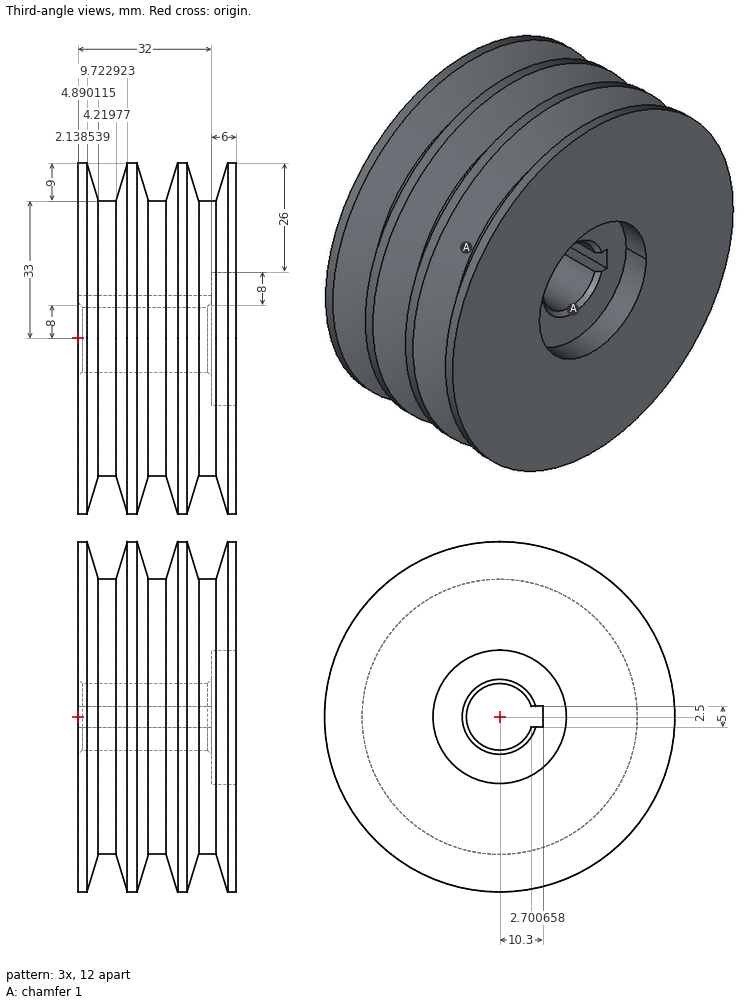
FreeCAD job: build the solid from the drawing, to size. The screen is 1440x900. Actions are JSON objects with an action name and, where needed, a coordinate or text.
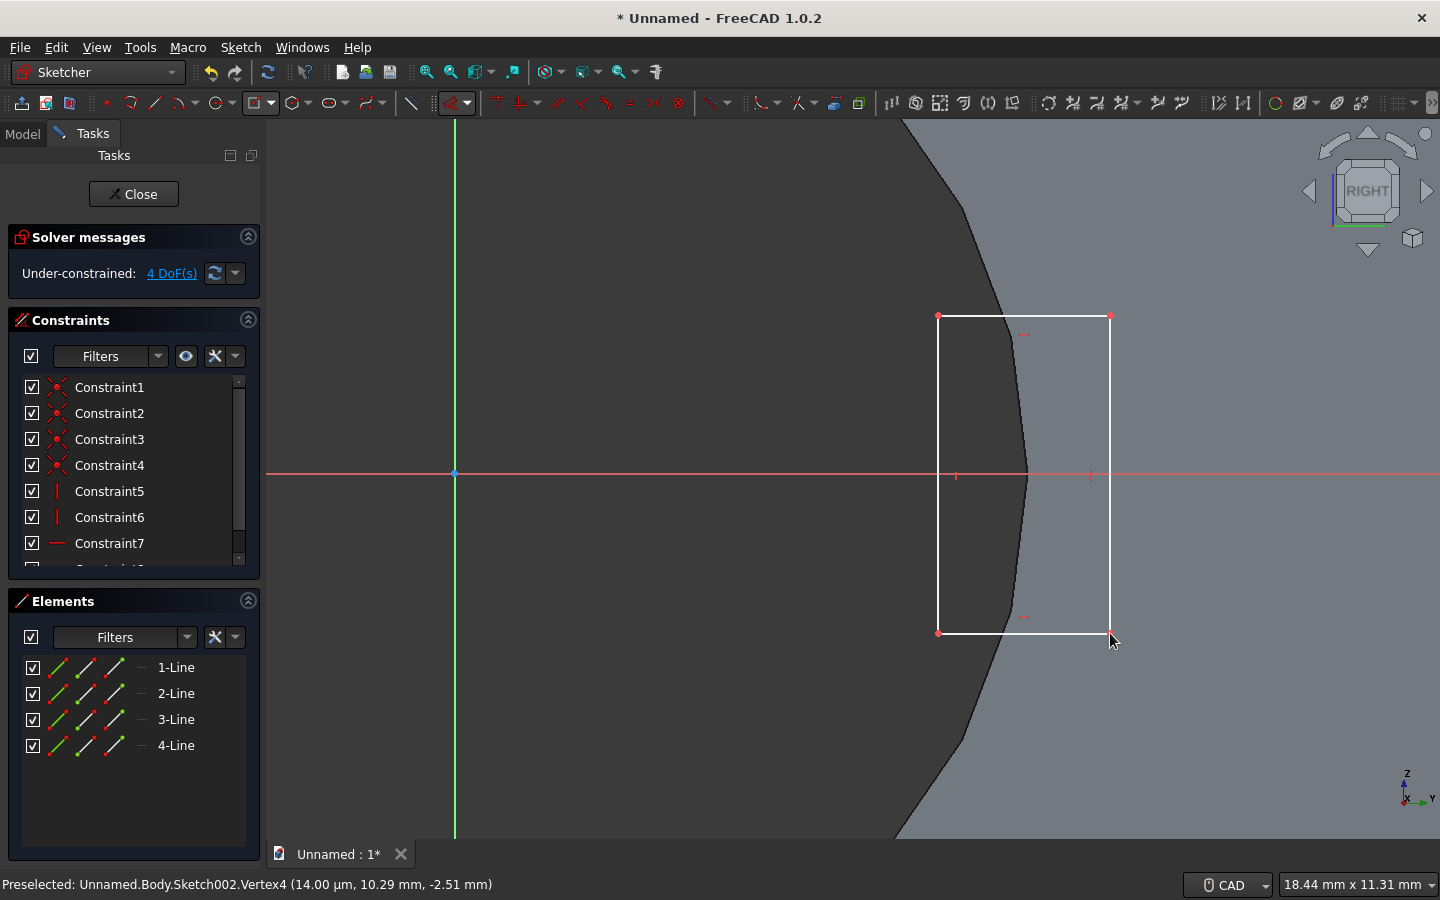
{"action": "key", "text": "d"}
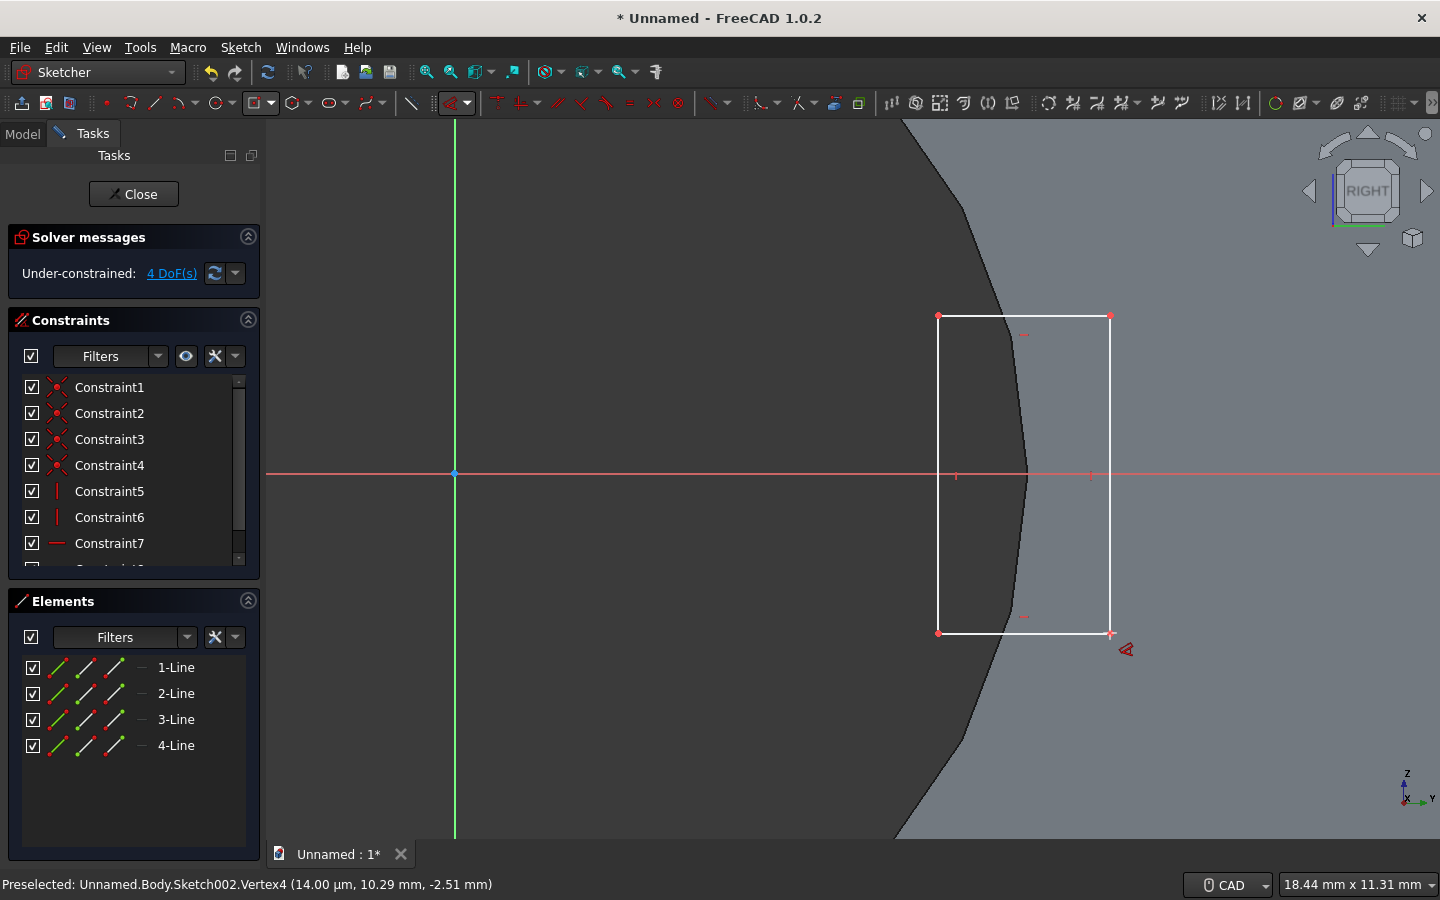
{"action": "left_click", "coordinate": [938, 411]}
{"action": "left_click", "coordinate": [972, 402]}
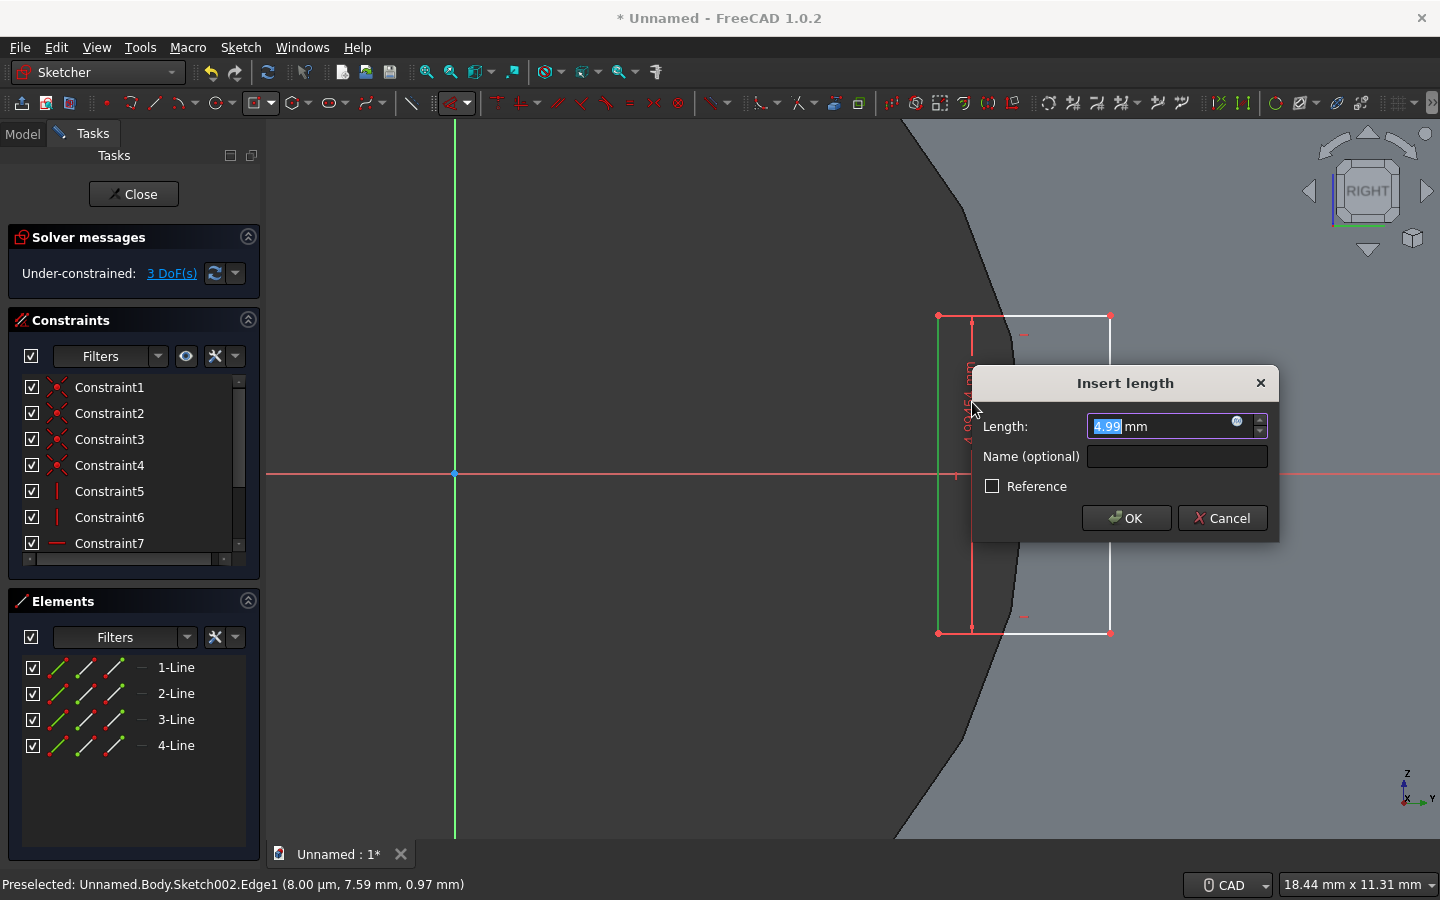
{"action": "type", "text": "5"}
{"action": "key", "text": "Return"}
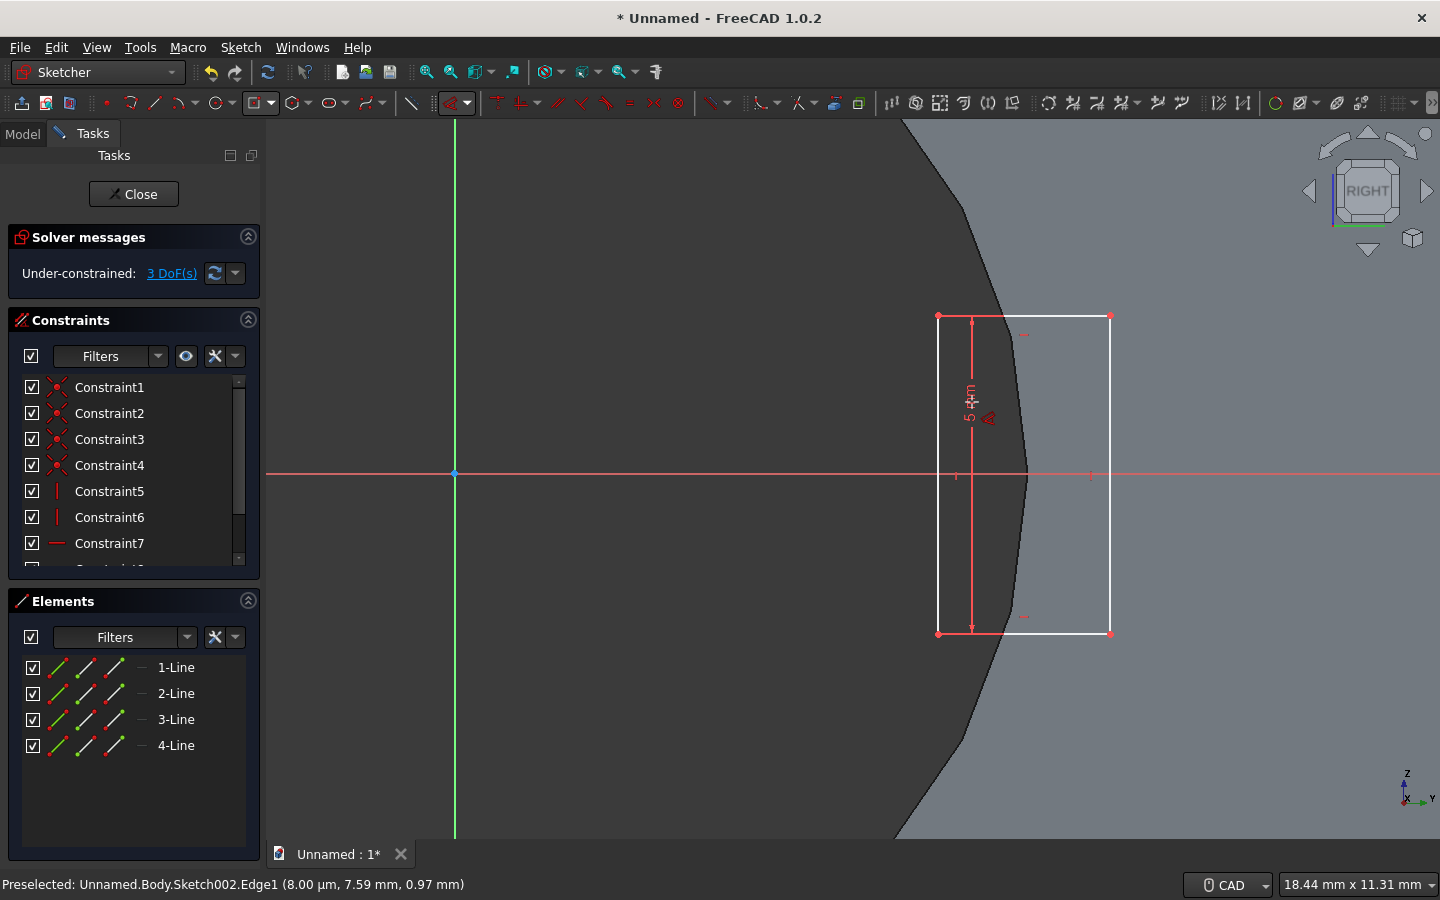
{"action": "left_click", "coordinate": [938, 316]}
{"action": "left_click", "coordinate": [421, 395]}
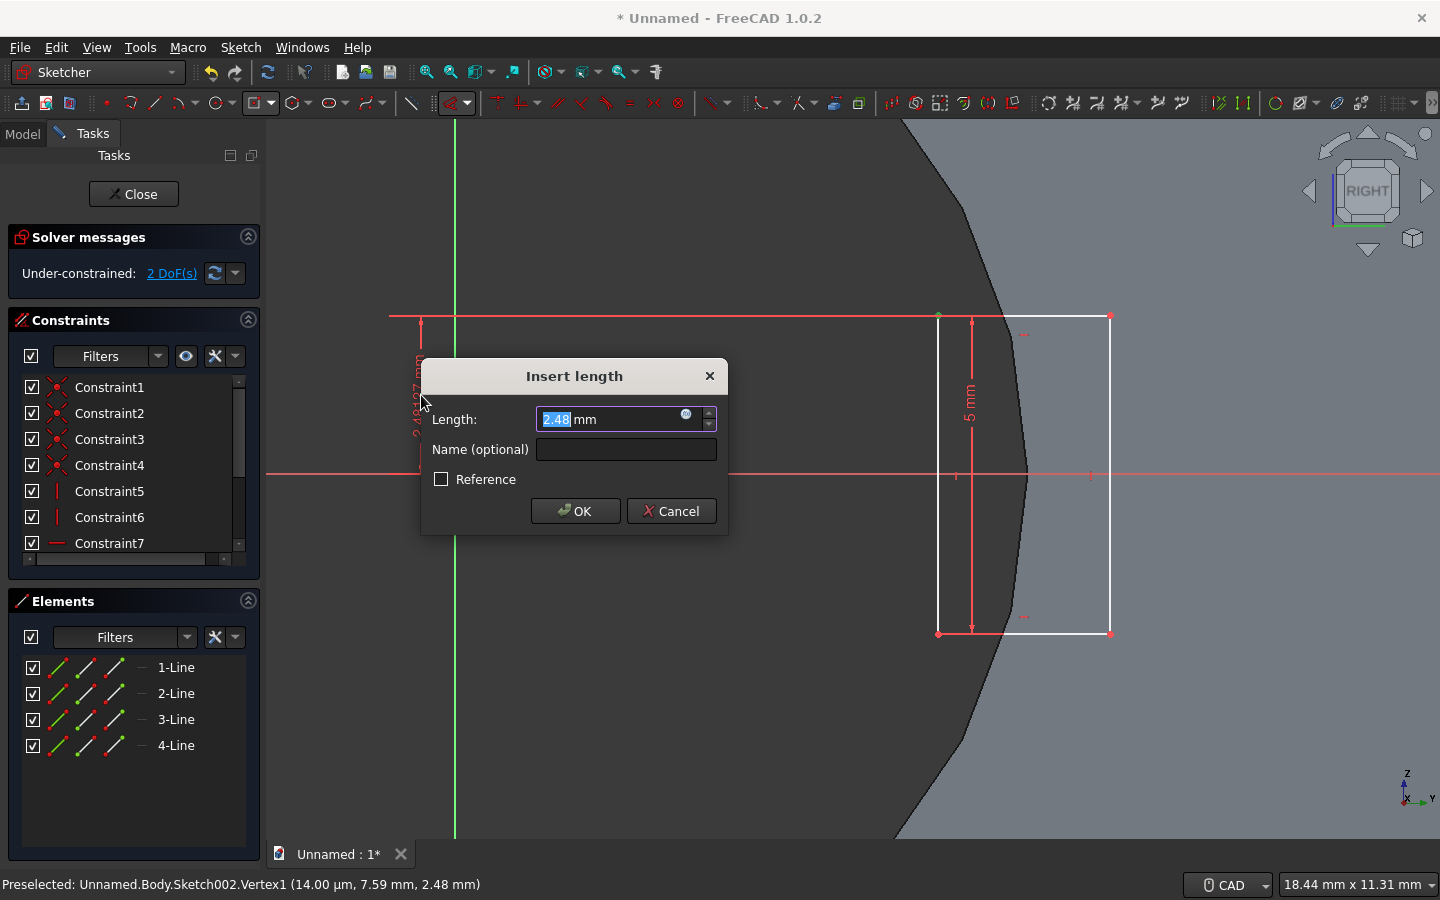
{"action": "type", "text": "2.5"}
{"action": "key", "text": "Return"}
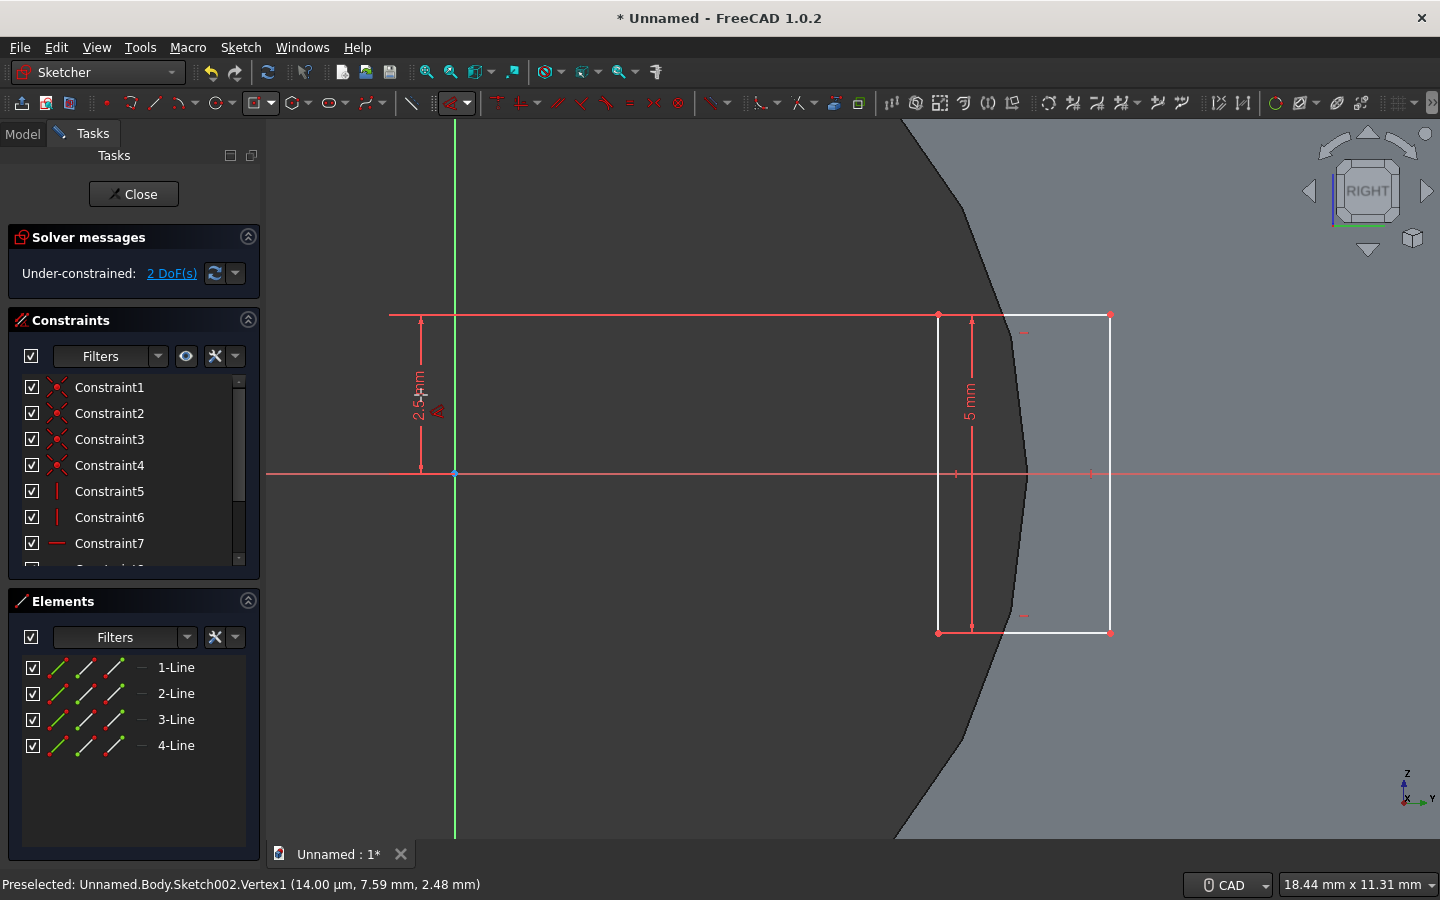
{"action": "left_click", "coordinate": [1110, 633]}
{"action": "left_click", "coordinate": [782, 667]}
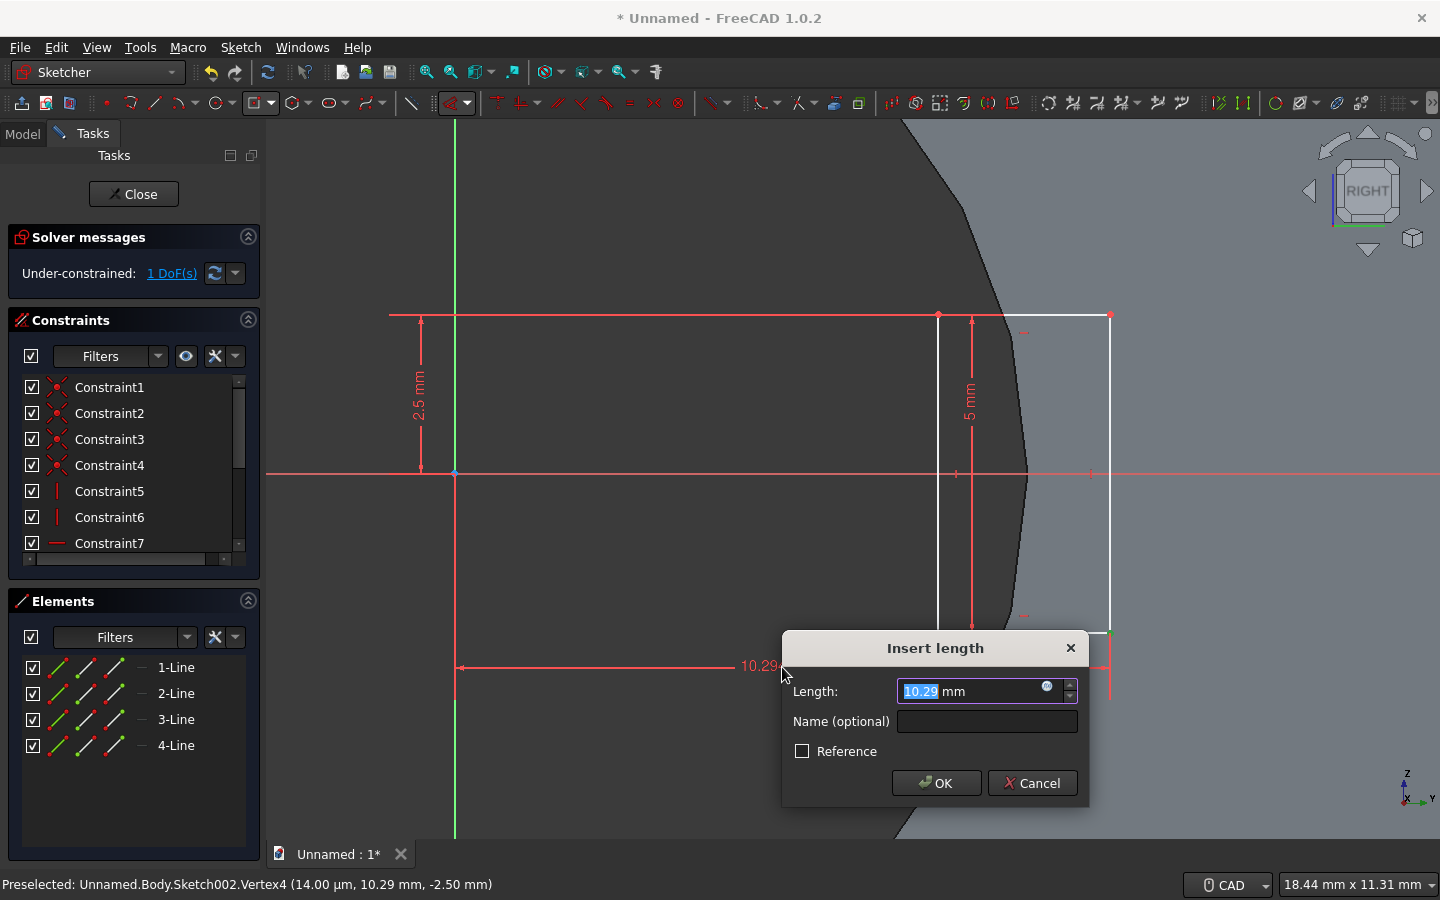
{"action": "type", "text": "10.3"}
{"action": "key", "text": "Return"}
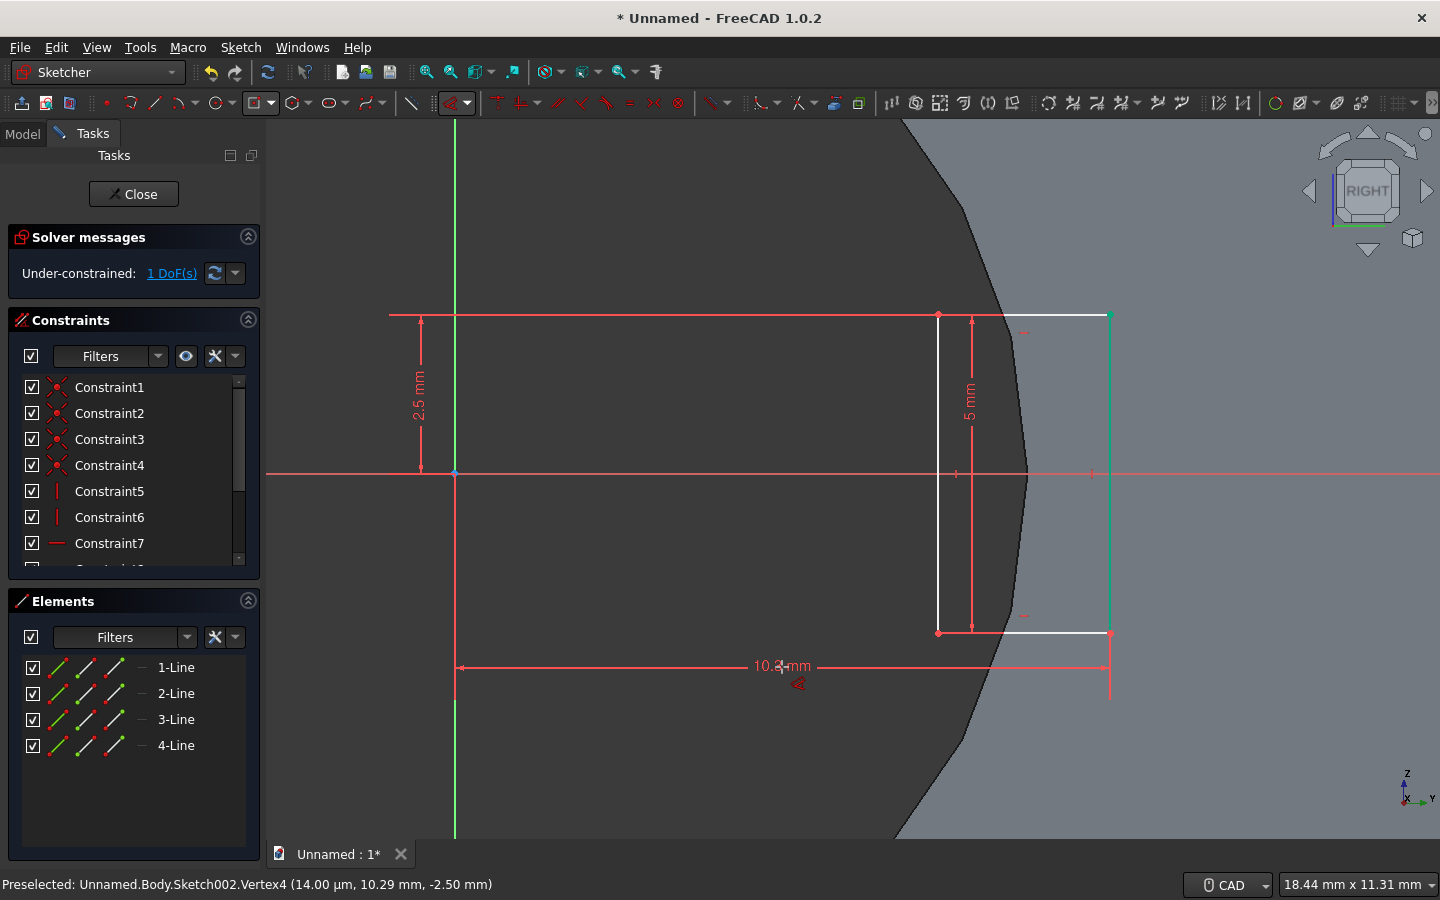
{"action": "left_click", "coordinate": [990, 633]}
{"action": "left_click", "coordinate": [1024, 667]}